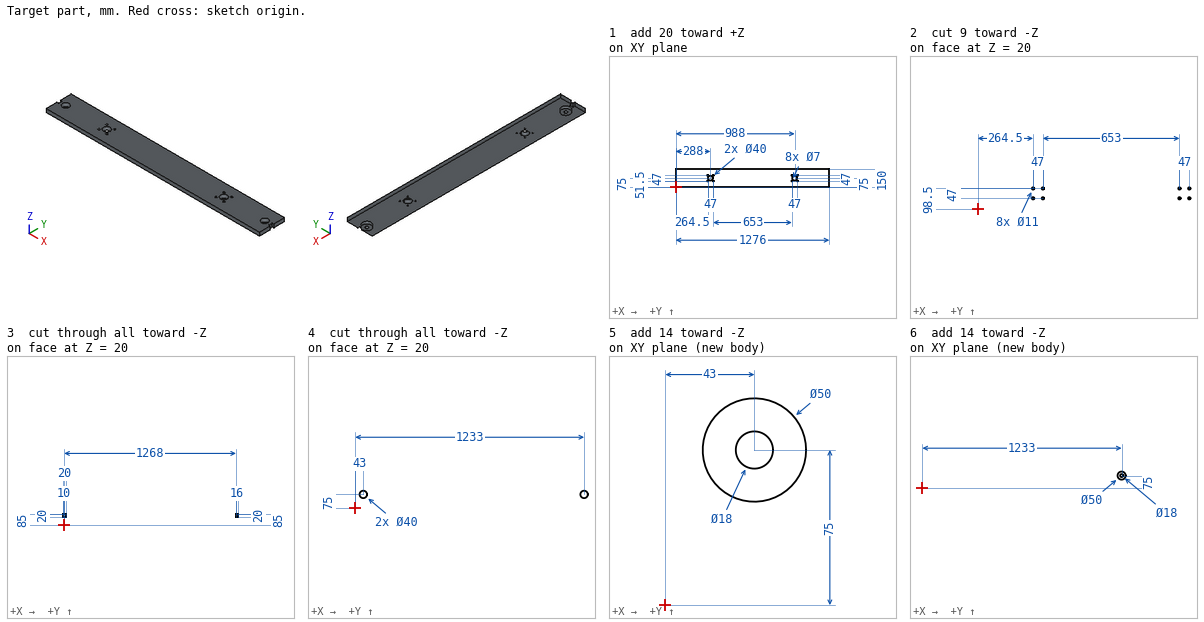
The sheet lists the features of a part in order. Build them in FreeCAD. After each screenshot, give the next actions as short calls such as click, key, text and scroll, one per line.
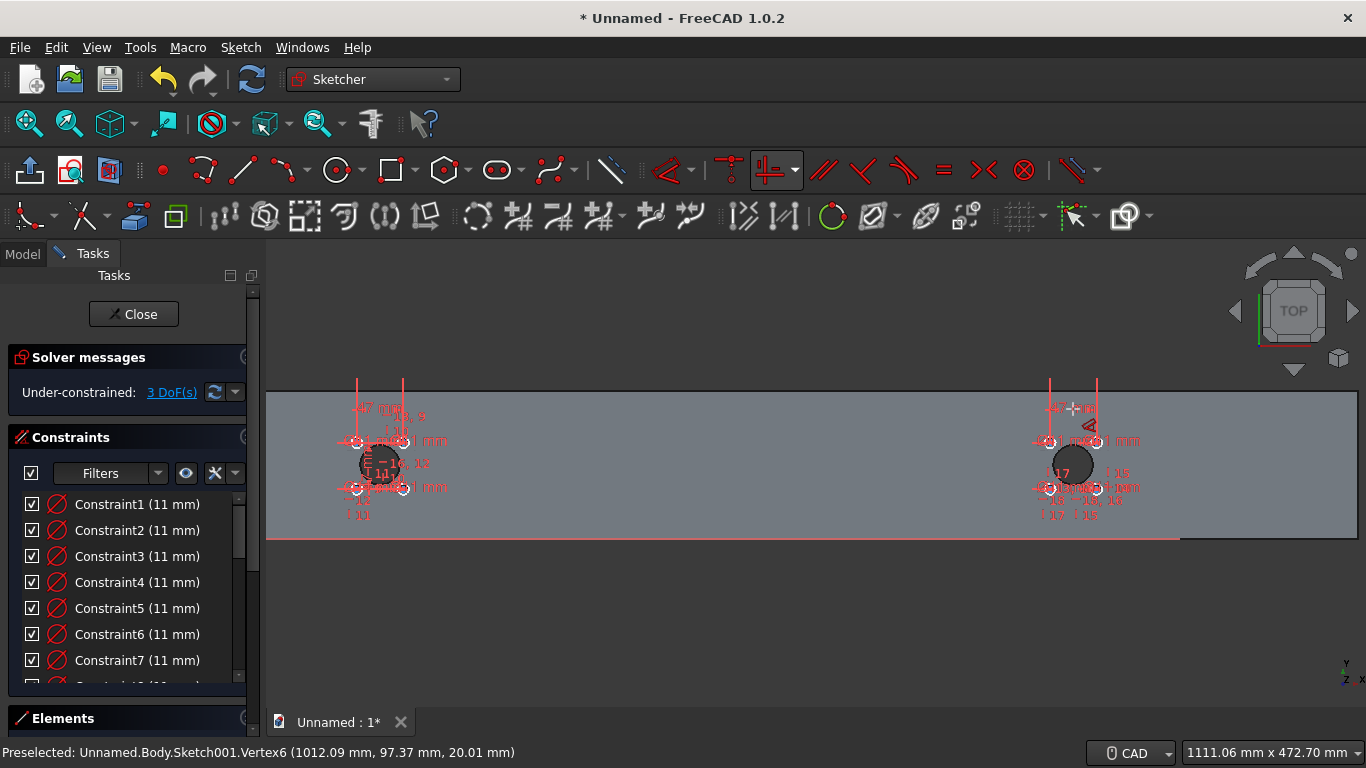
click(357, 443)
click(391, 513)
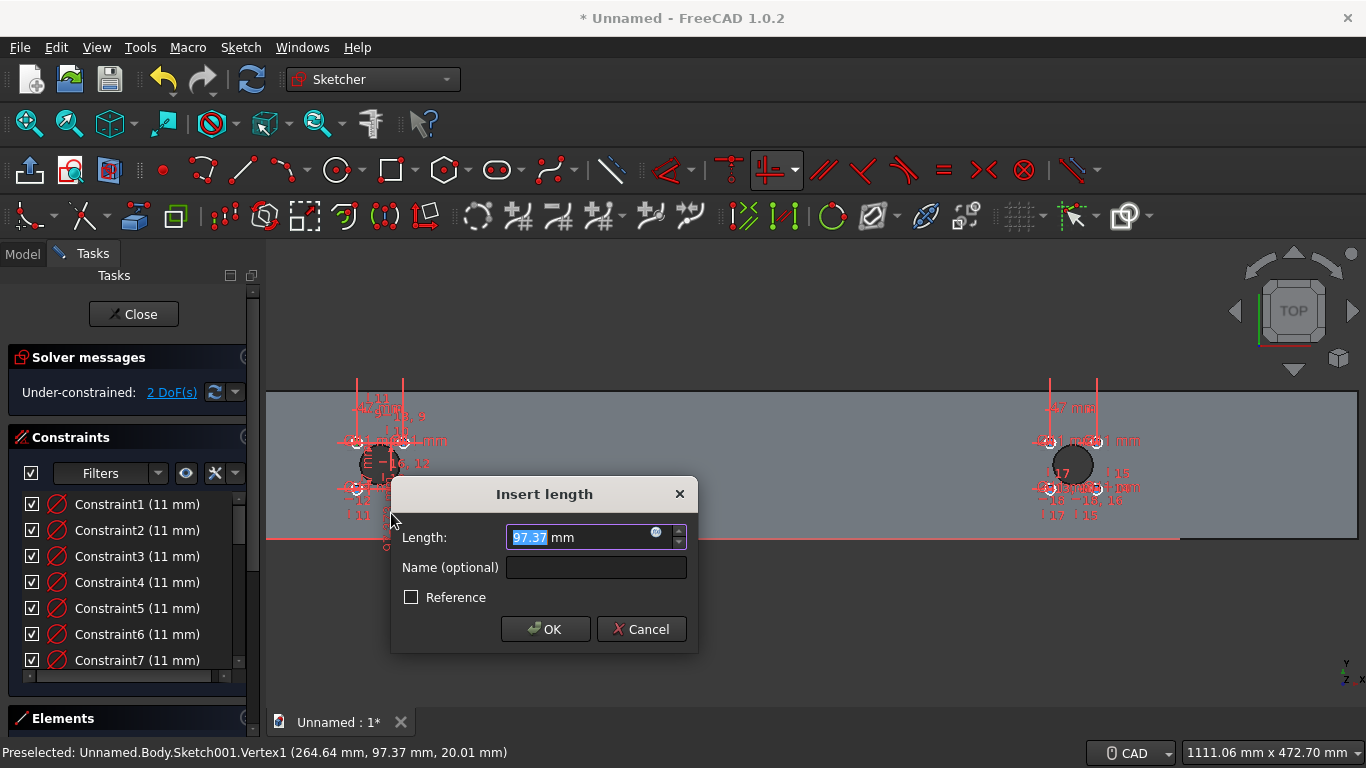
text(98.5)
key(Return)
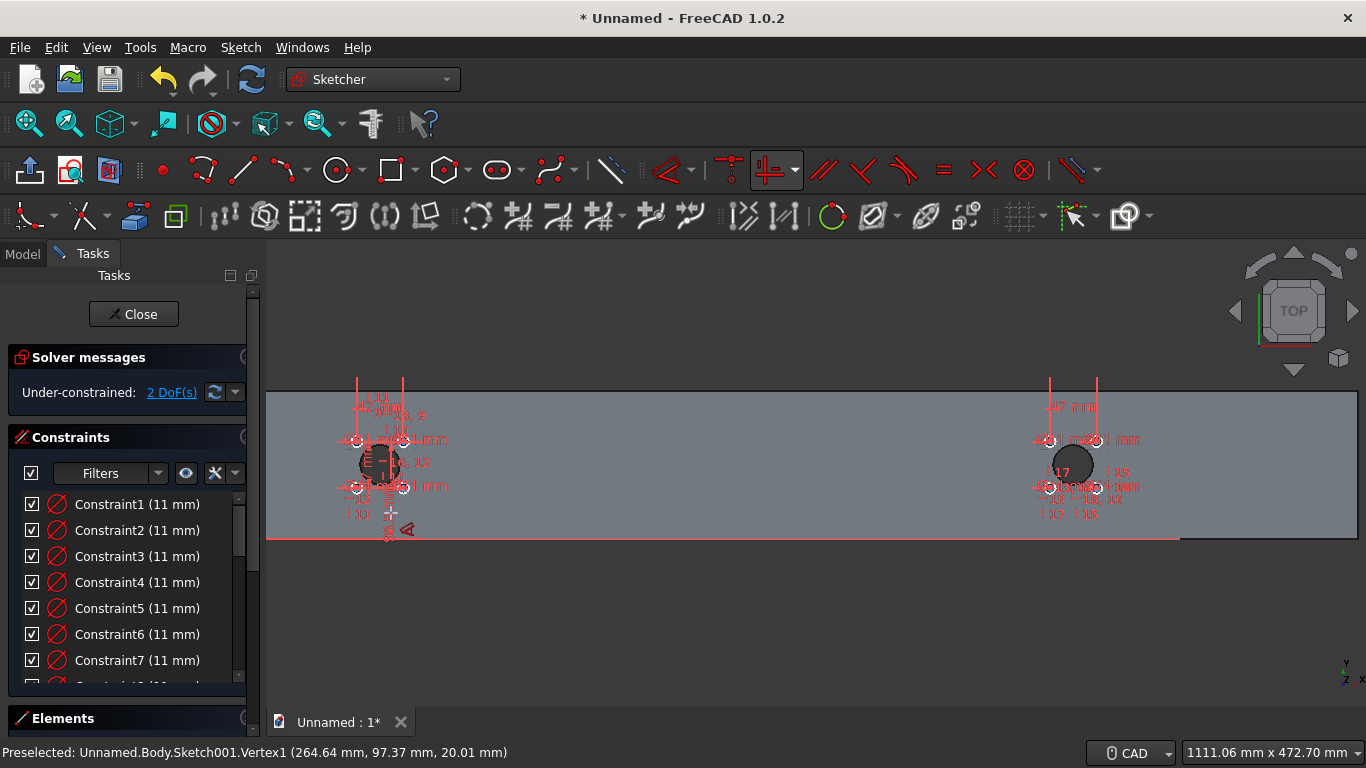
click(403, 442)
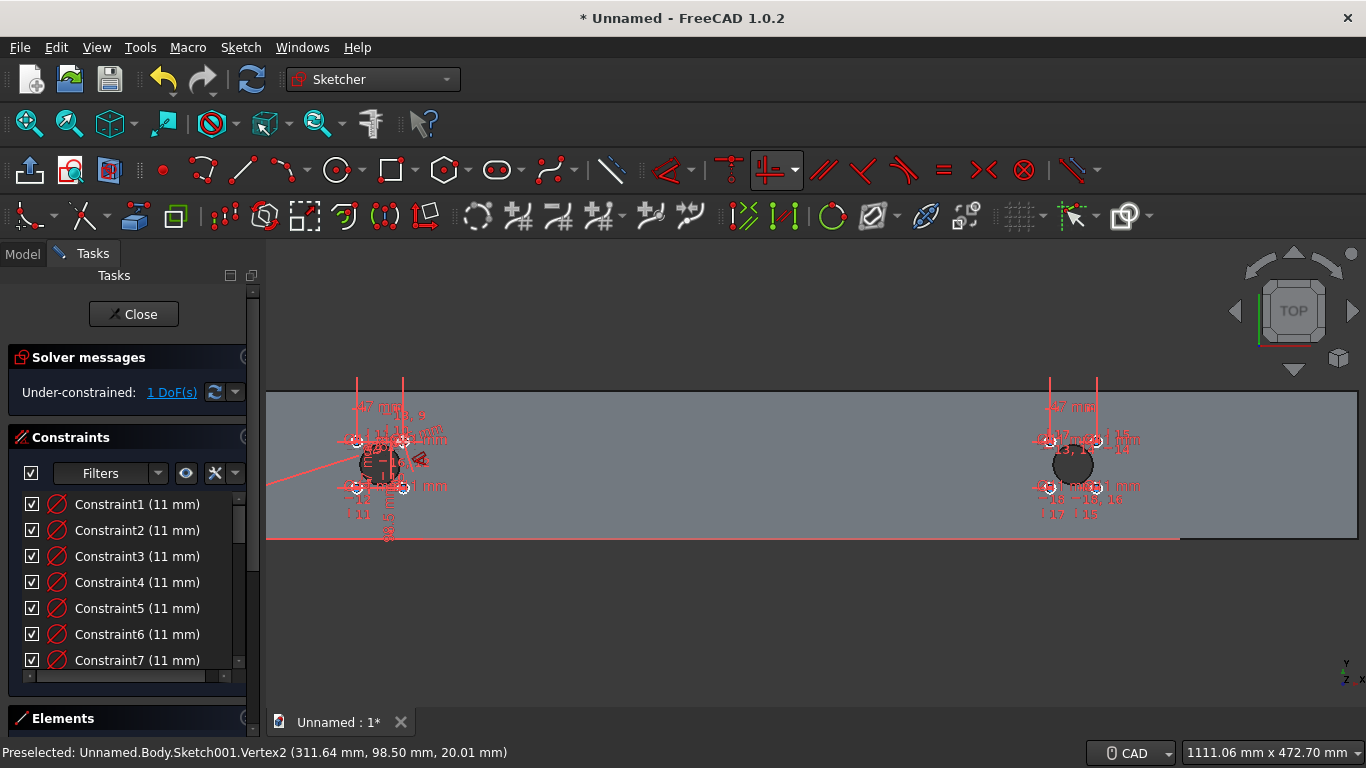
click(1050, 442)
click(727, 408)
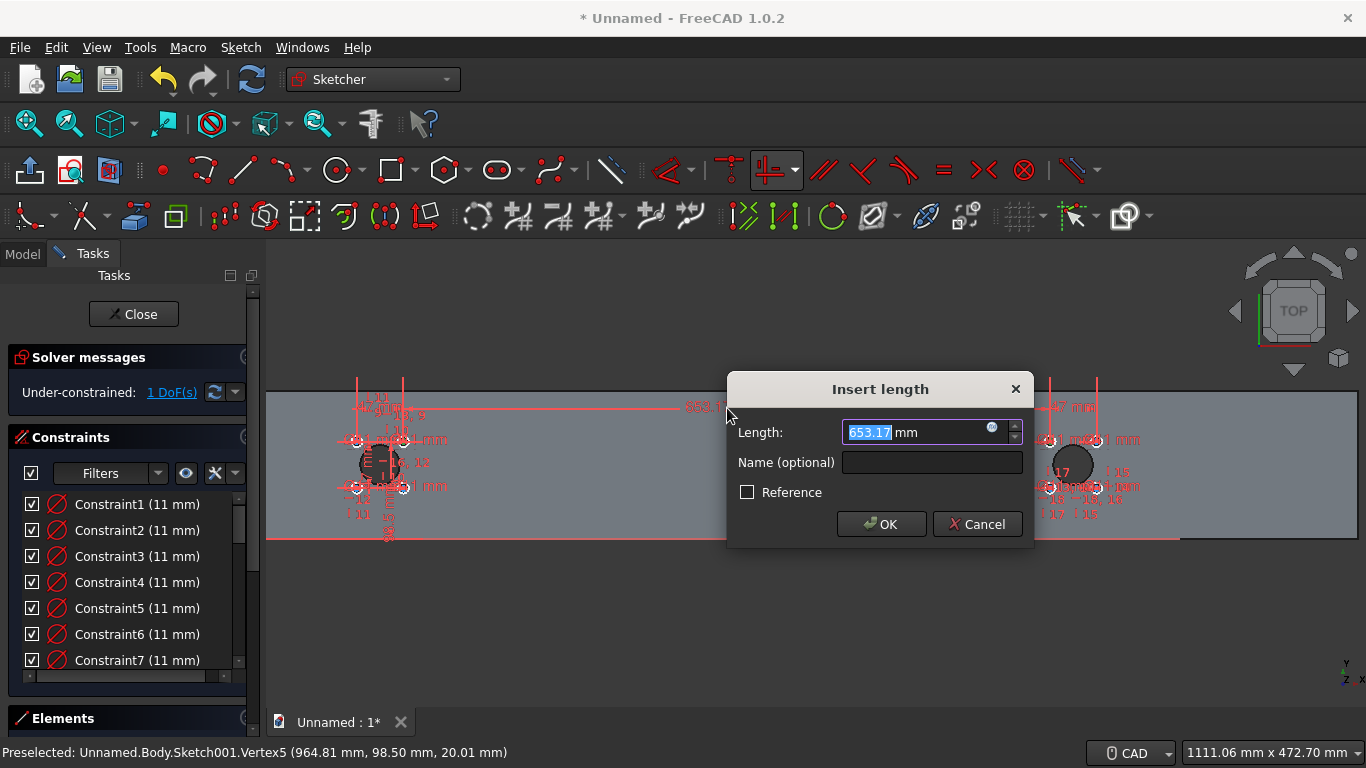
text(653)
key(Return)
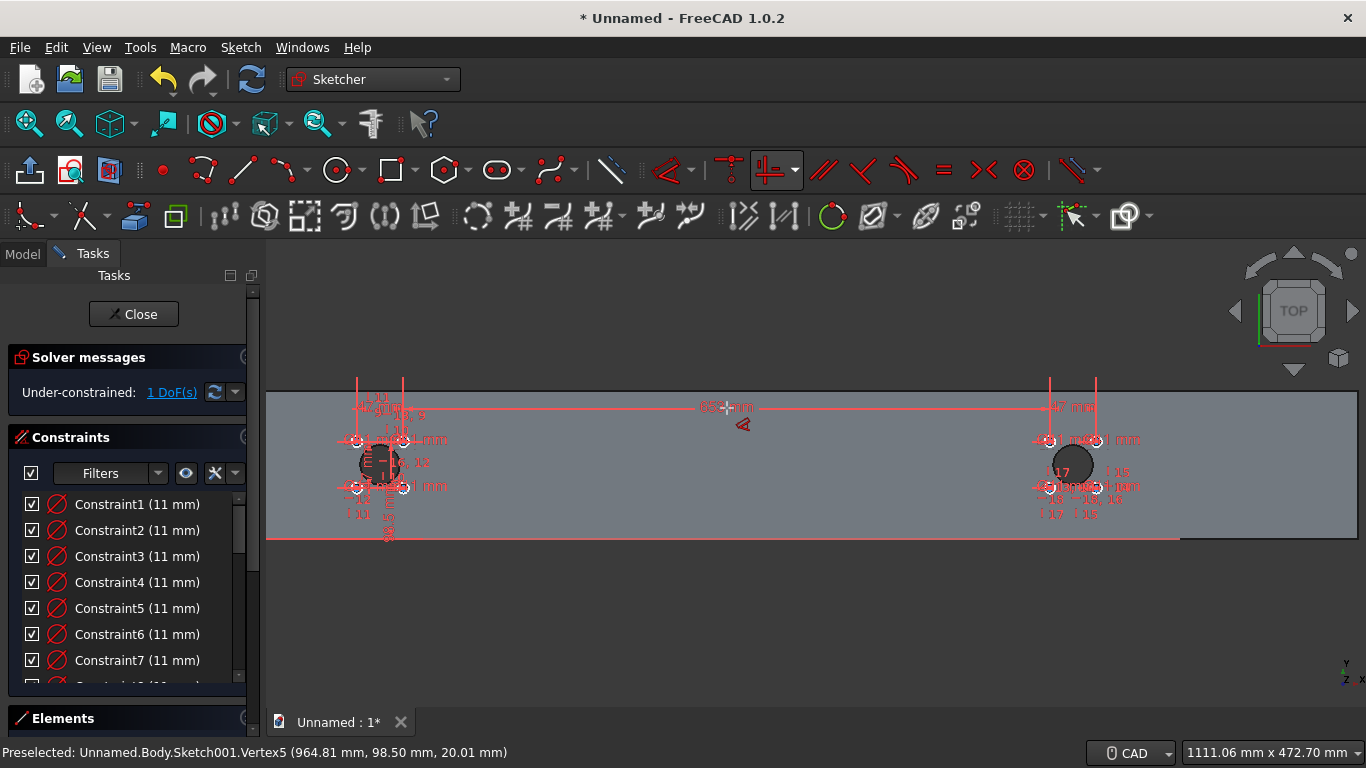
click(357, 442)
click(325, 573)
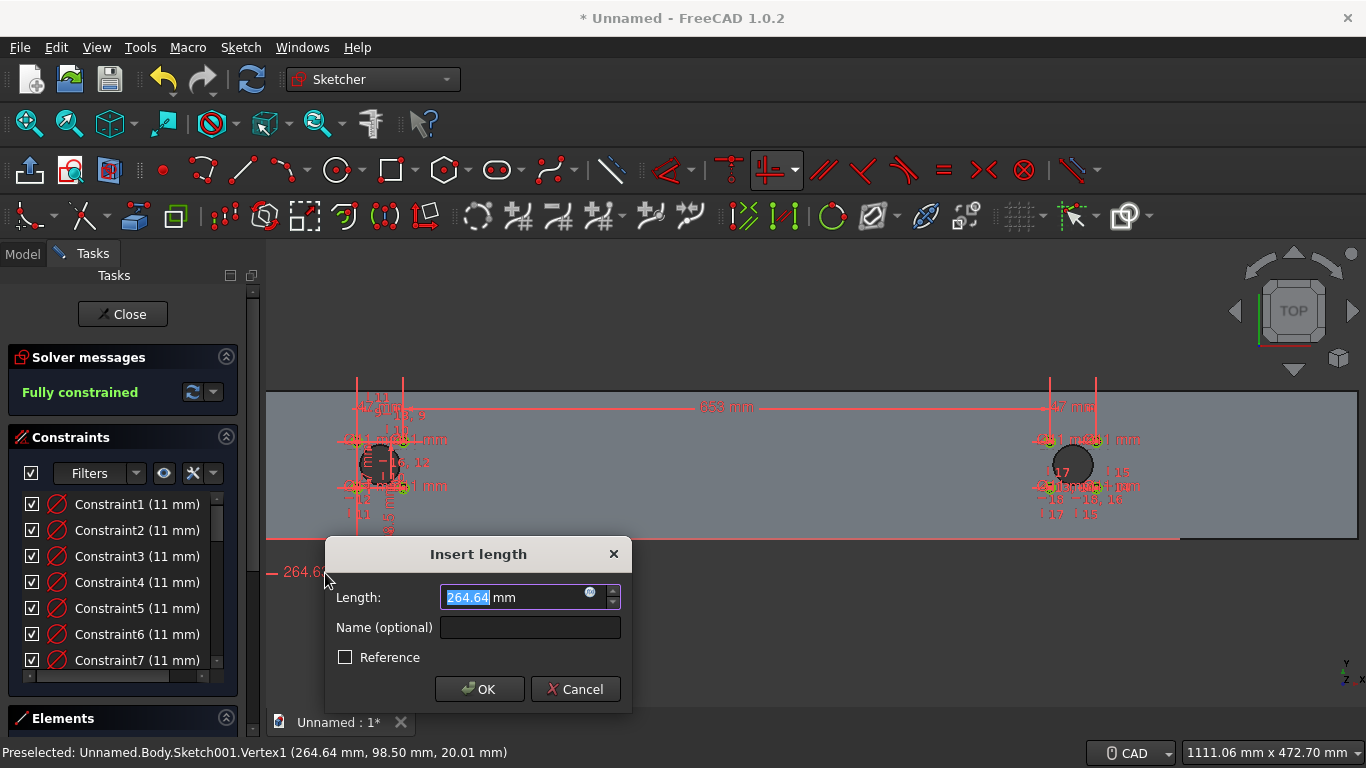
text(264.5)
key(Return)
key(Escape)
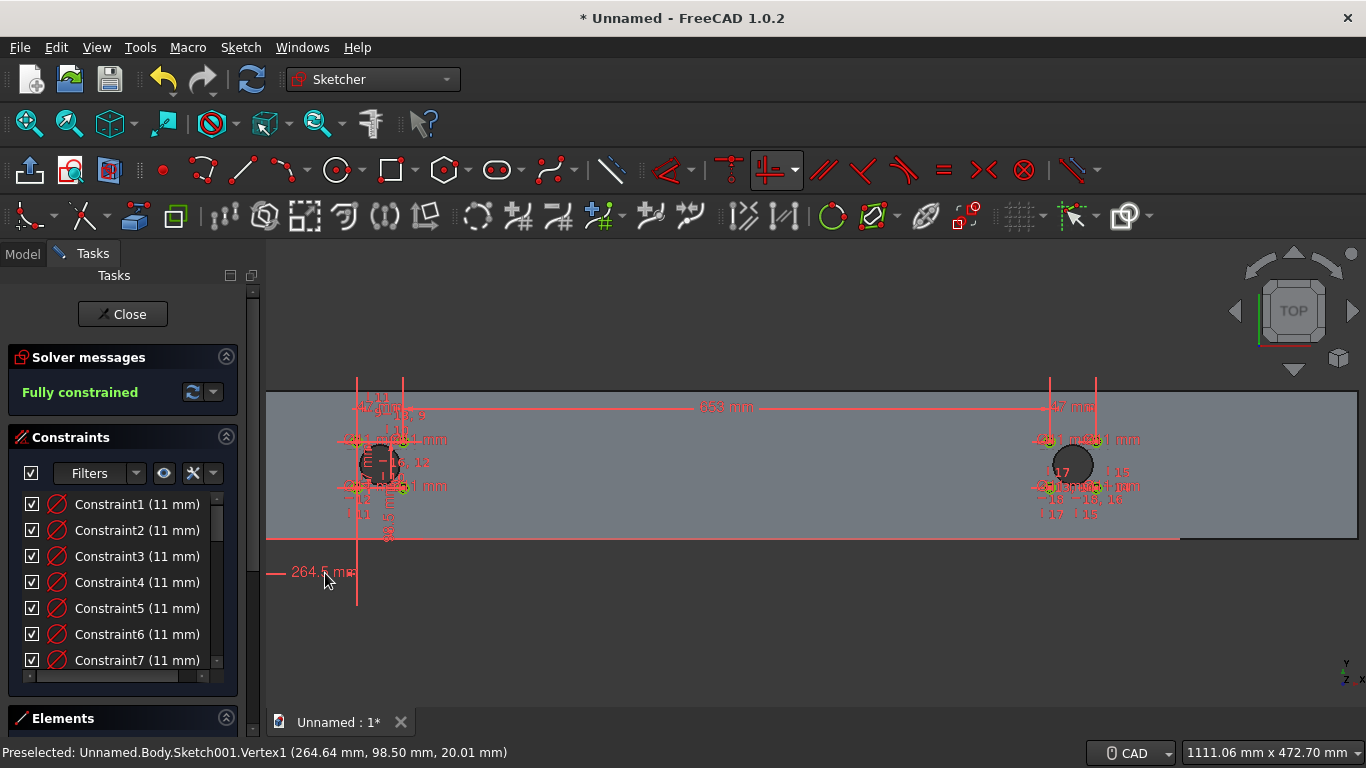
click(123, 314)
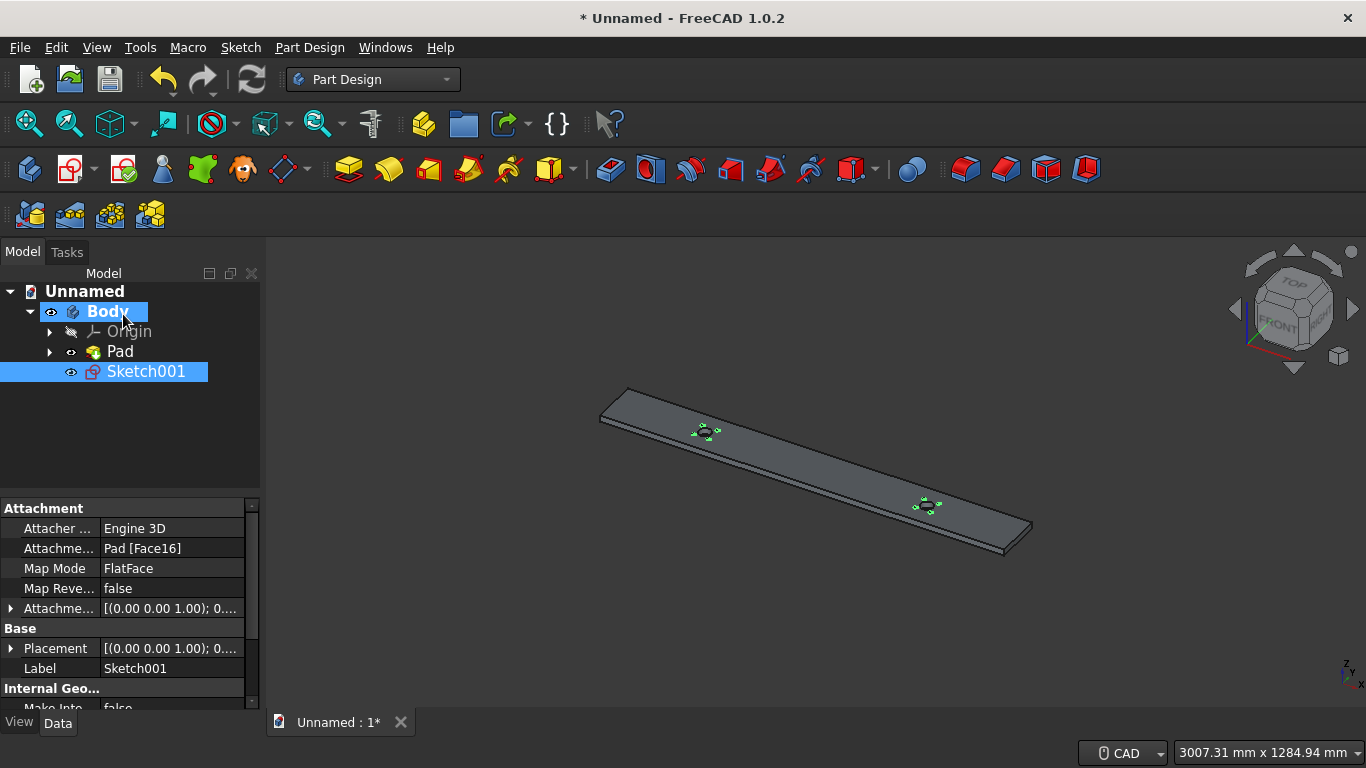
click(612, 170)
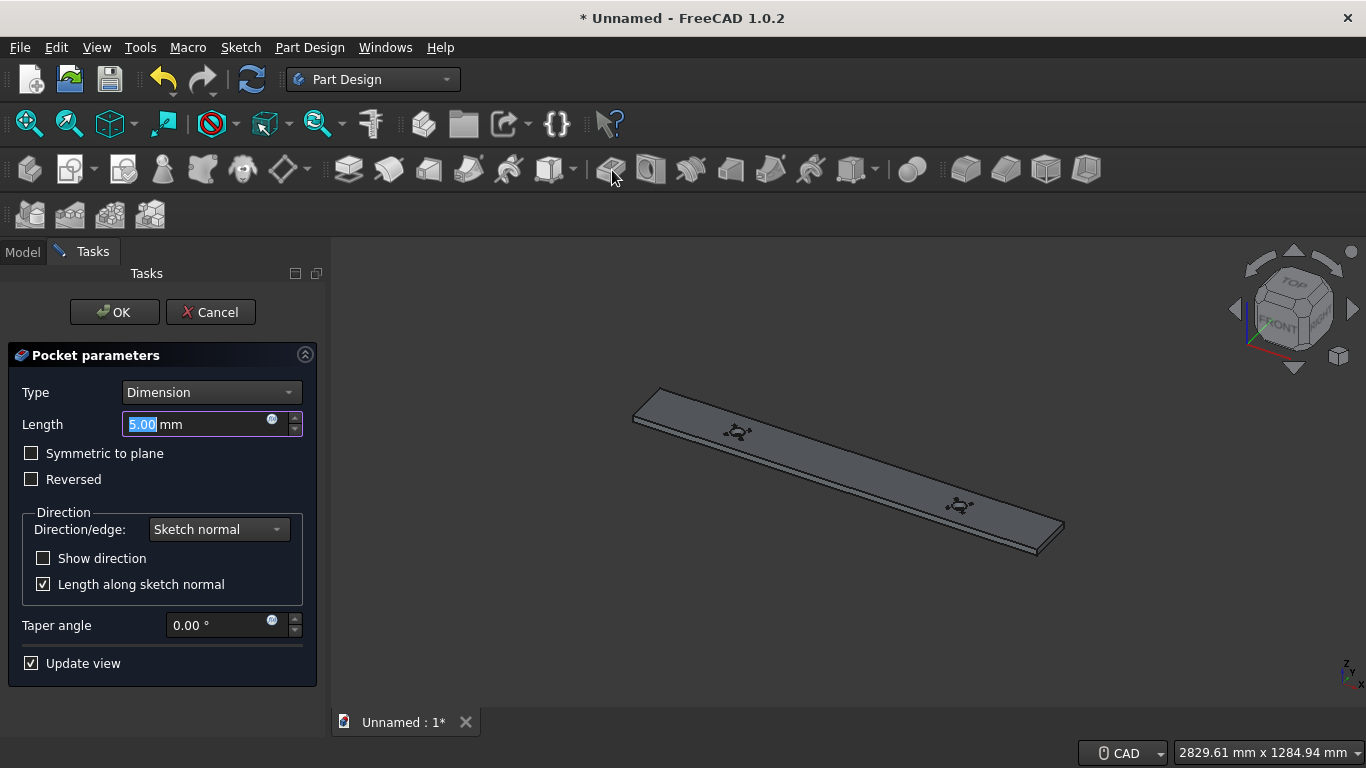
text(9)
key(Tab)